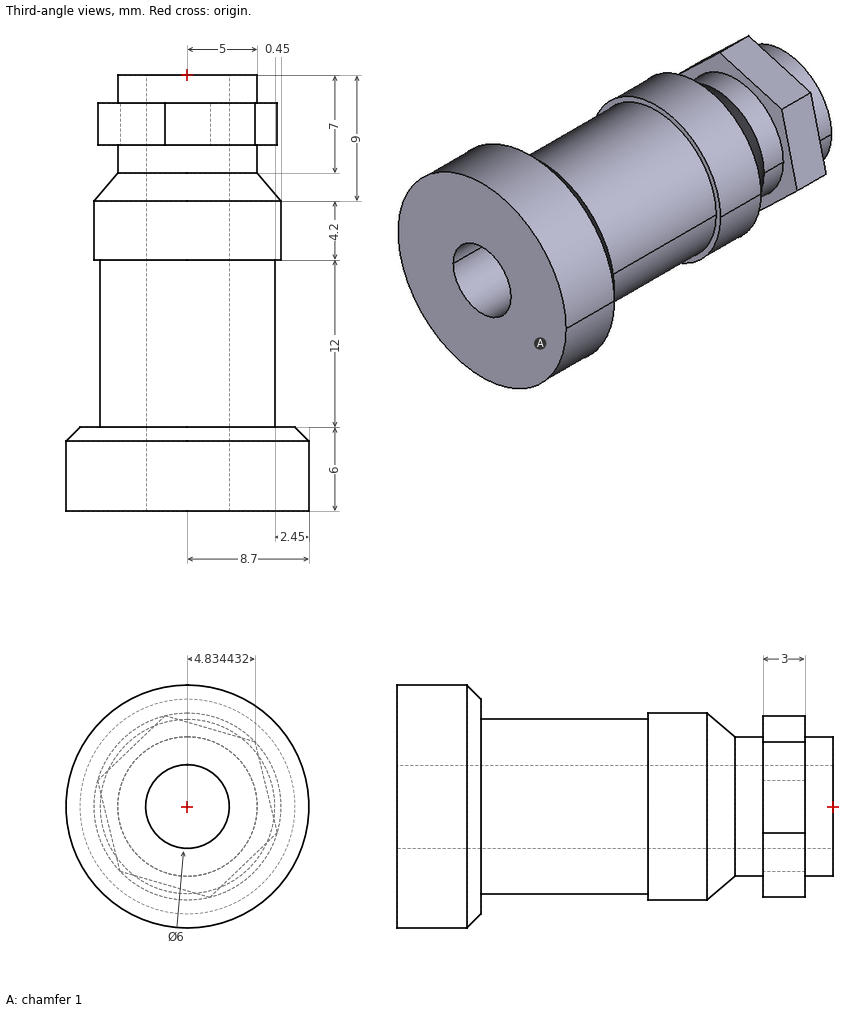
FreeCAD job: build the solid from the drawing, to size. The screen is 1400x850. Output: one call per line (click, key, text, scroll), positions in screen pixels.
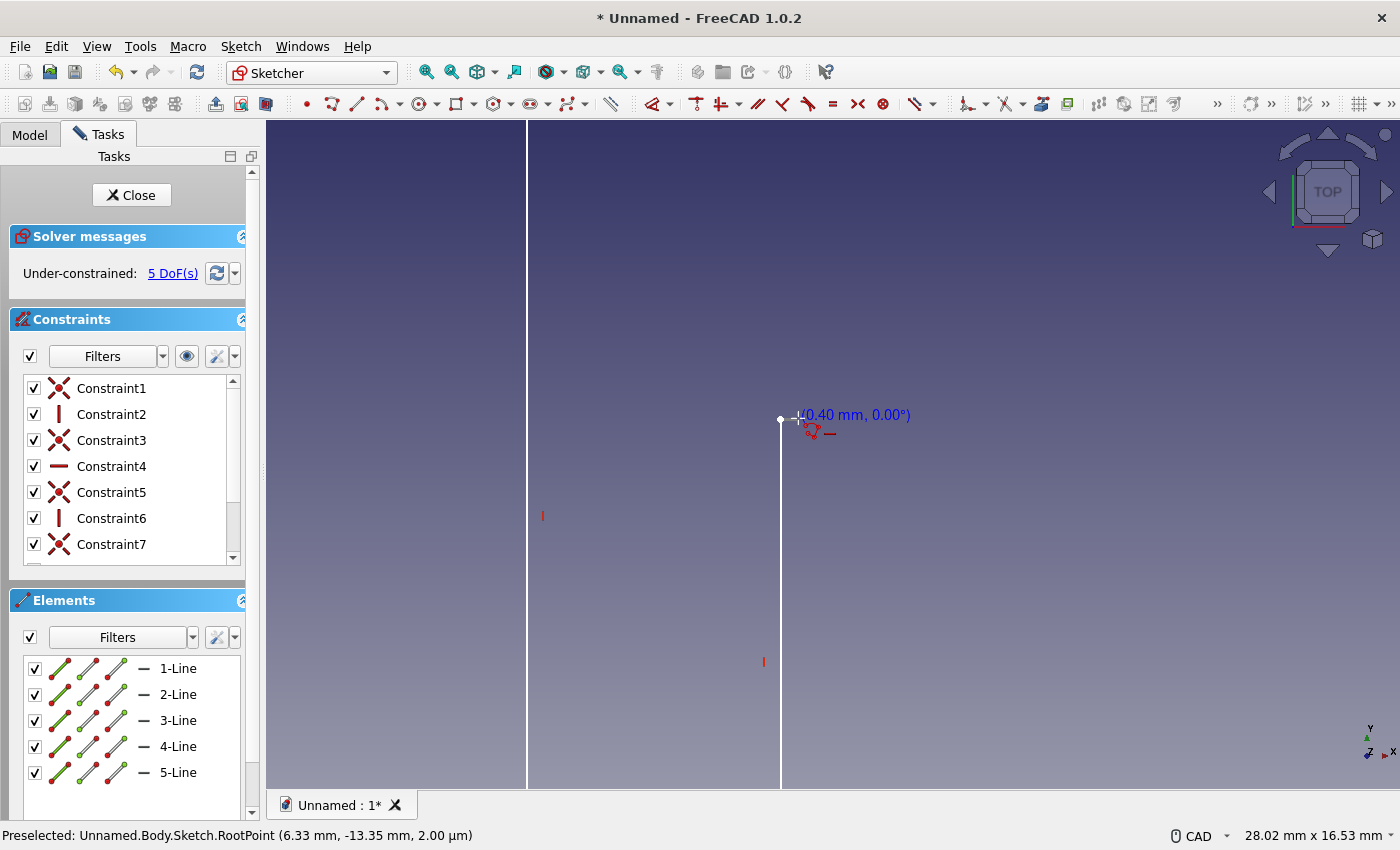
click(798, 417)
click(798, 247)
click(730, 166)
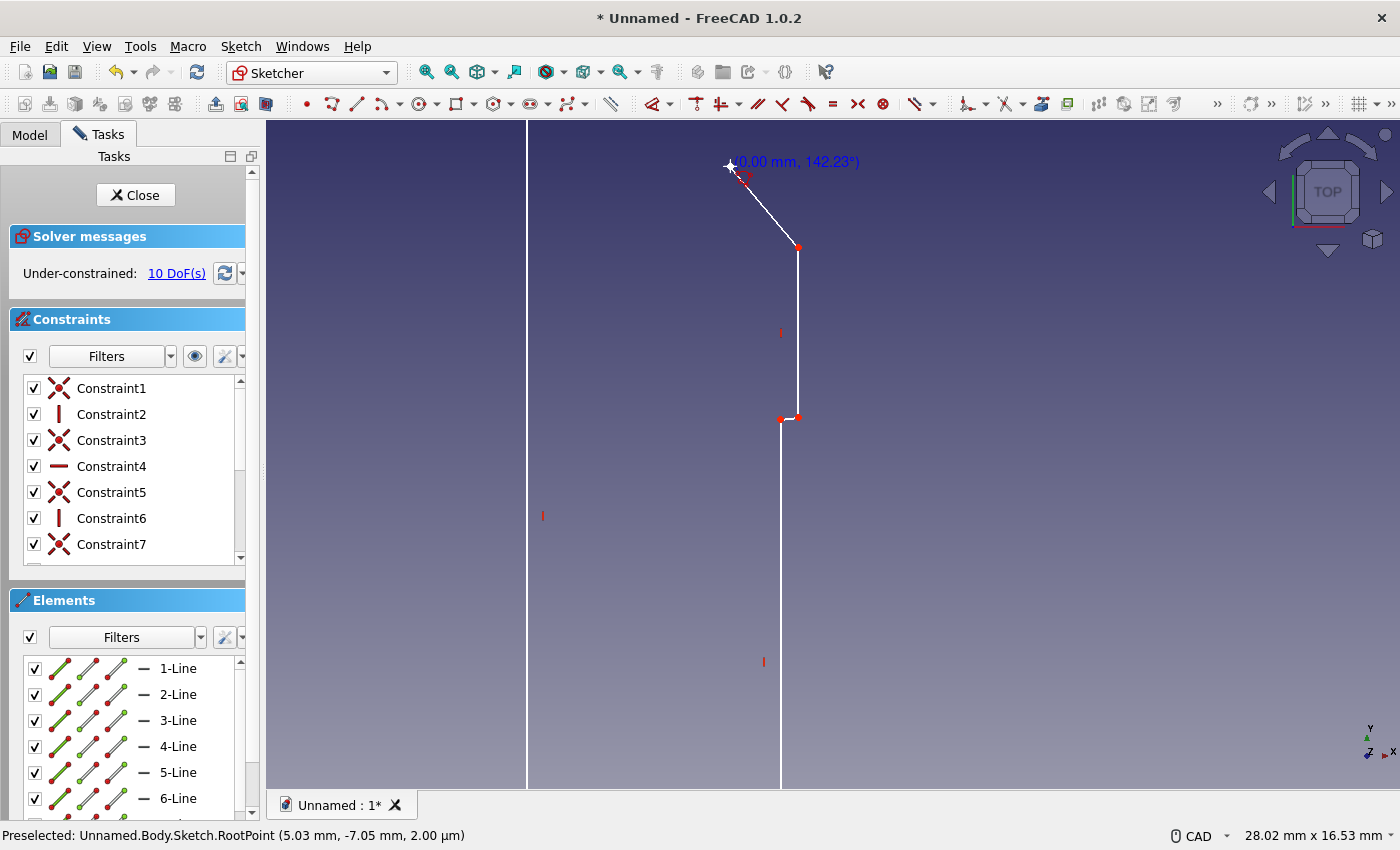
scroll(800, 420, down, 5)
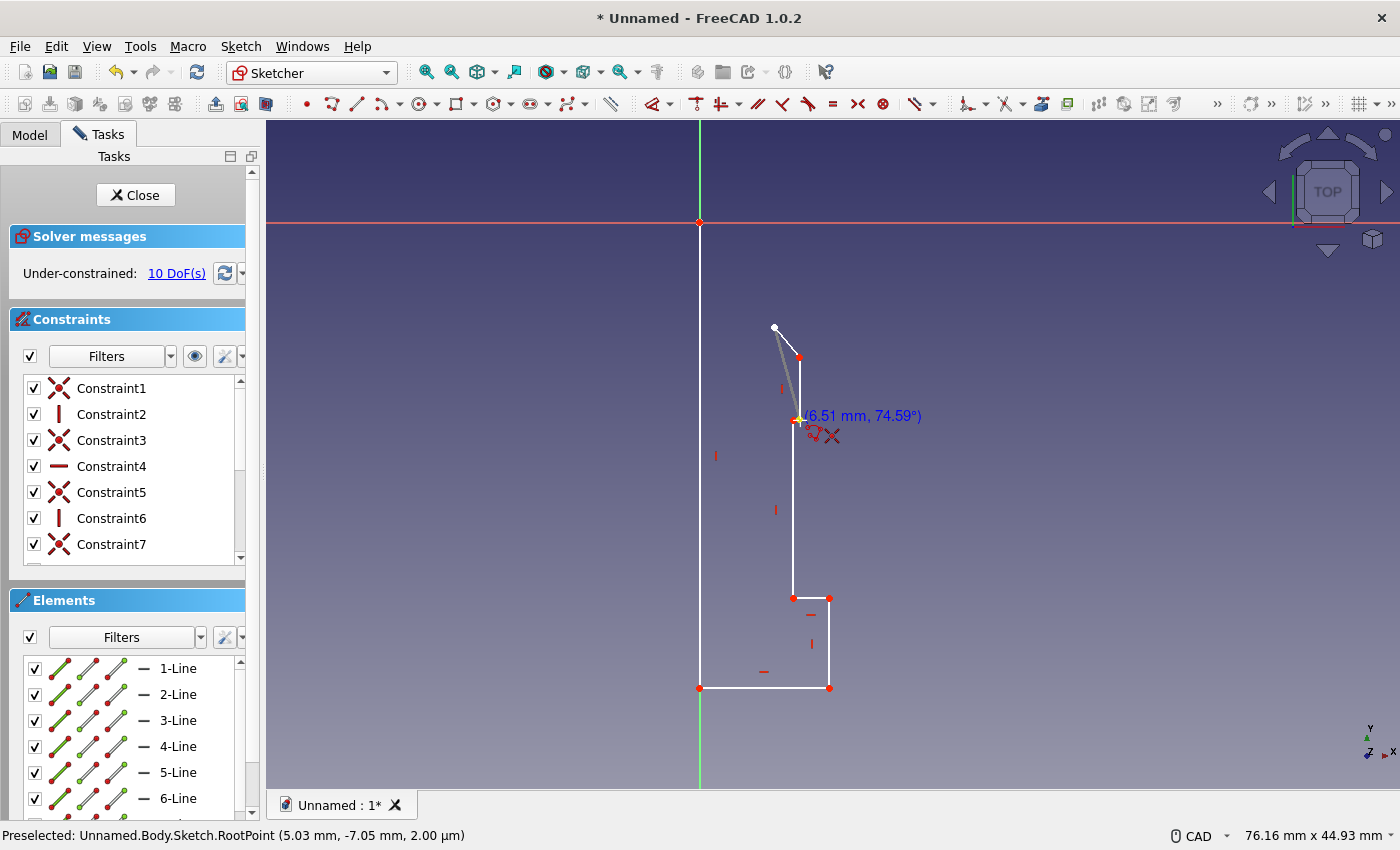
click(775, 232)
click(700, 223)
key(Escape)
key(Escape)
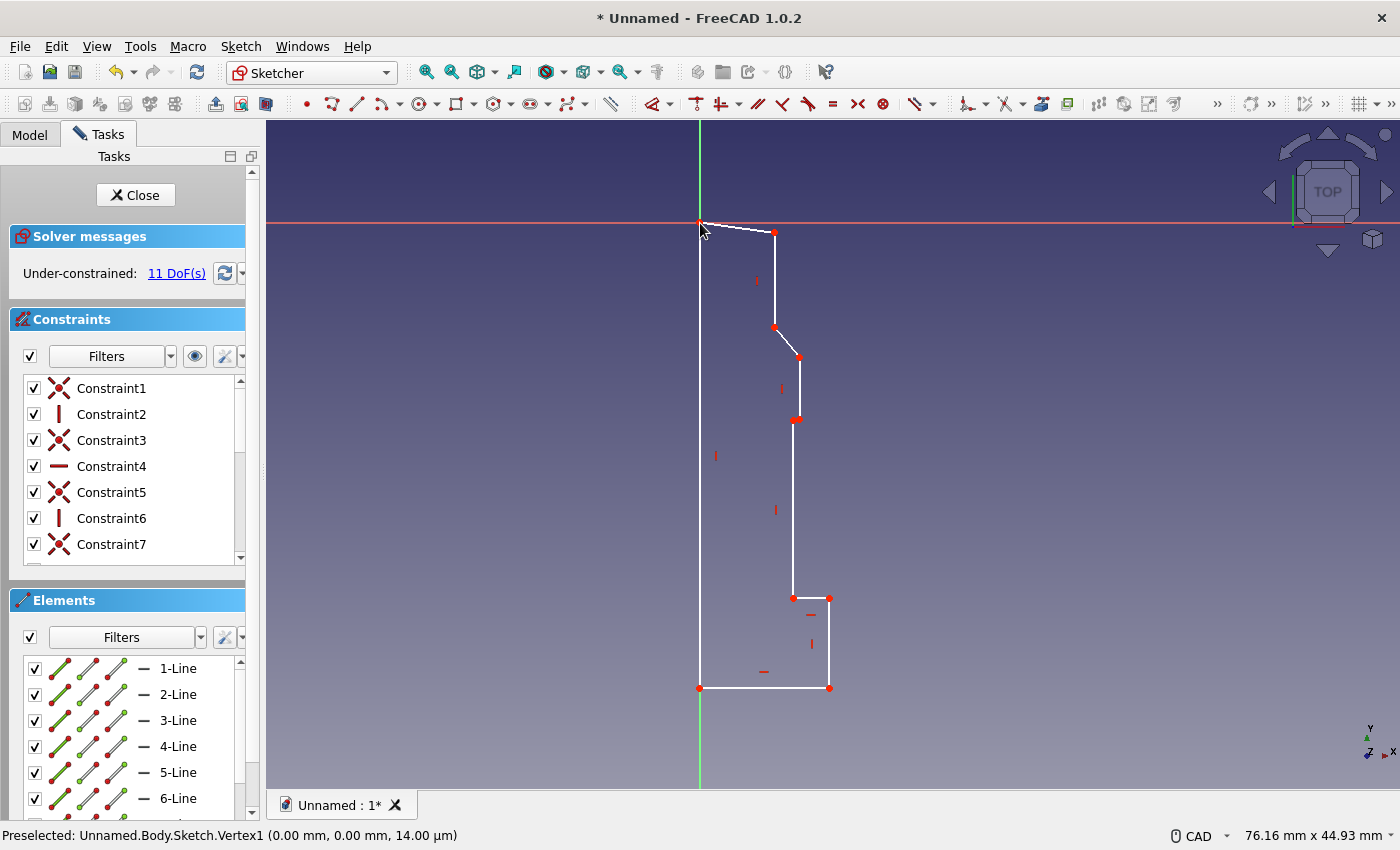
scroll(796, 420, up, 8)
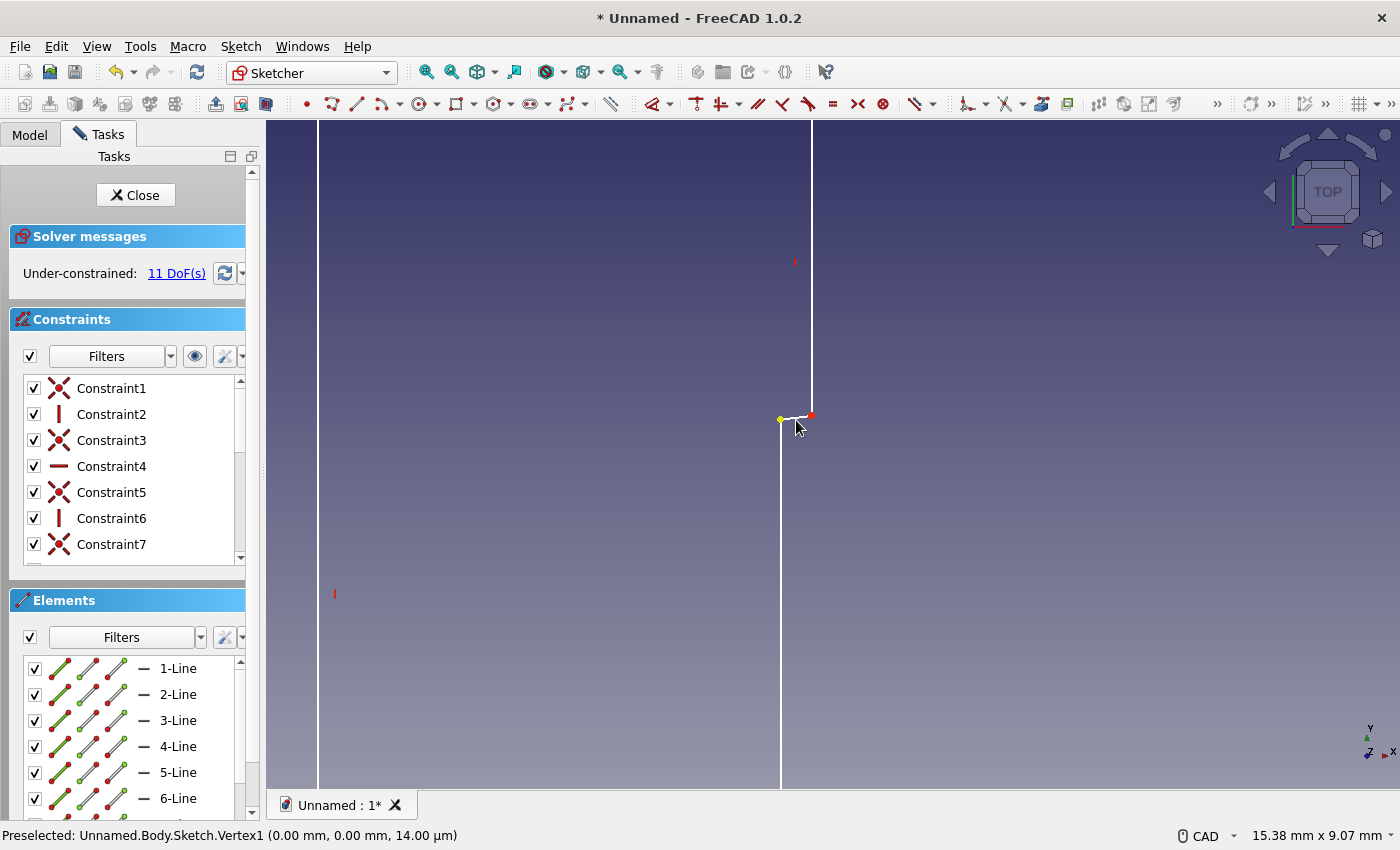
click(796, 418)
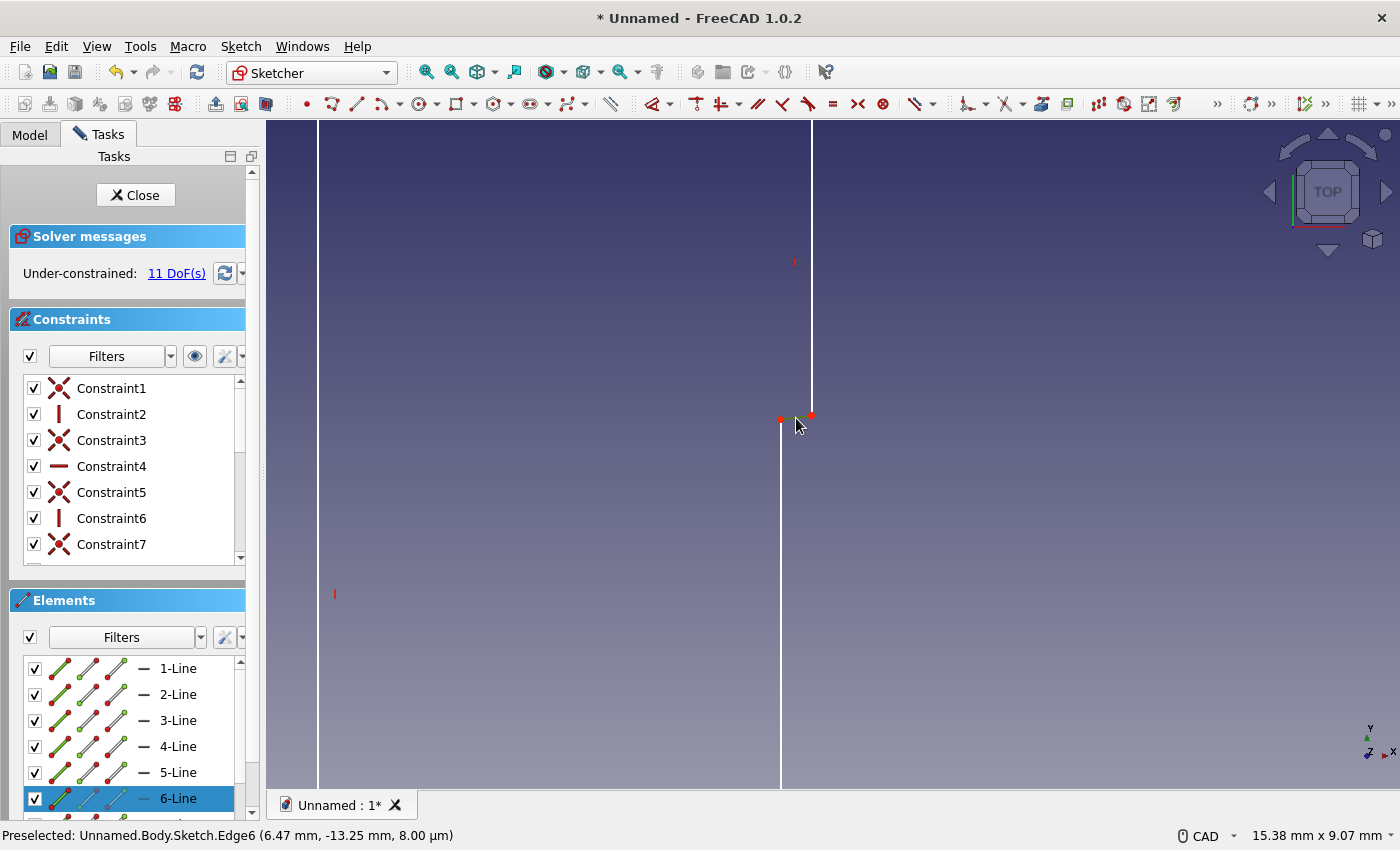
key(h)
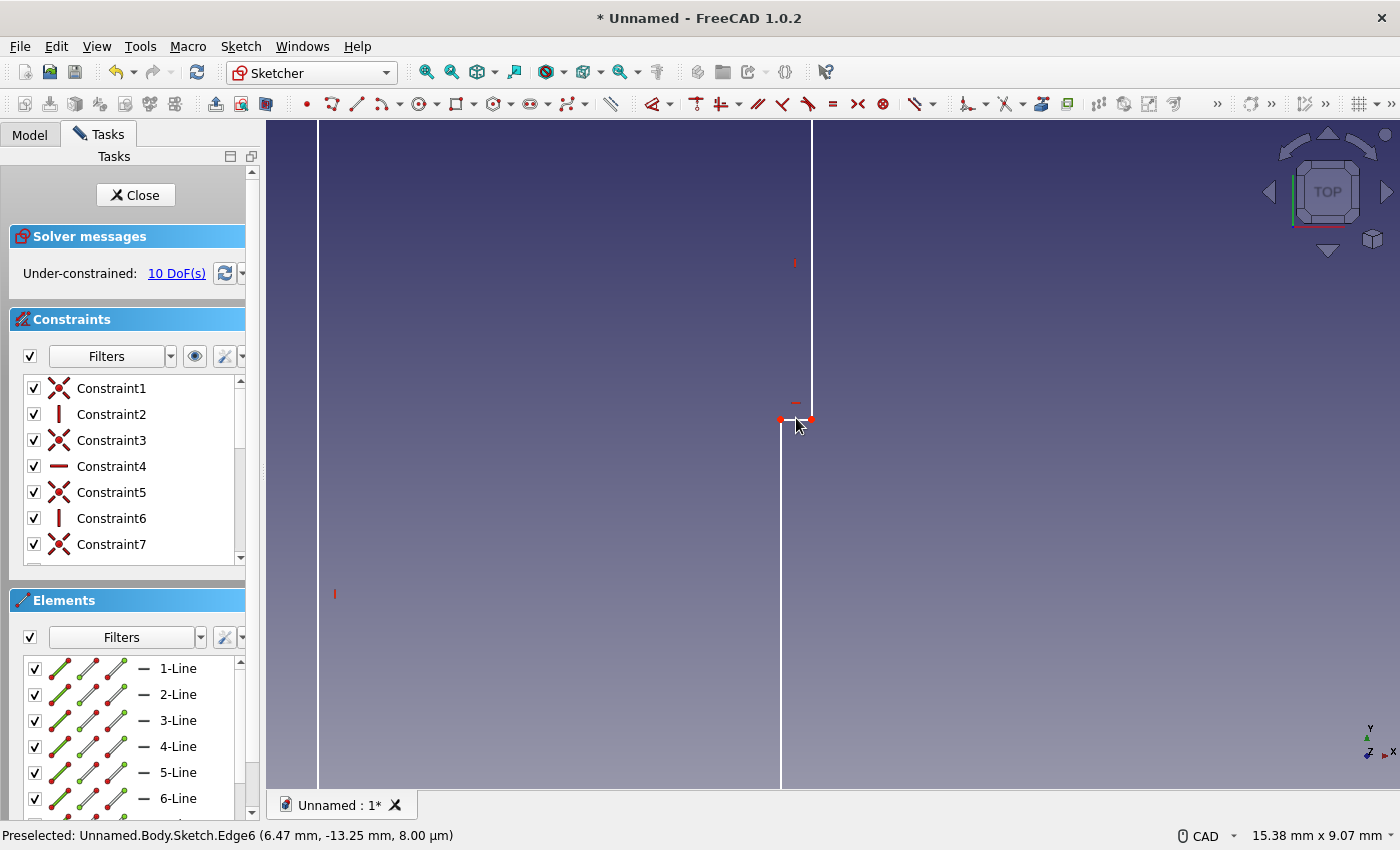
scroll(796, 420, down, 8)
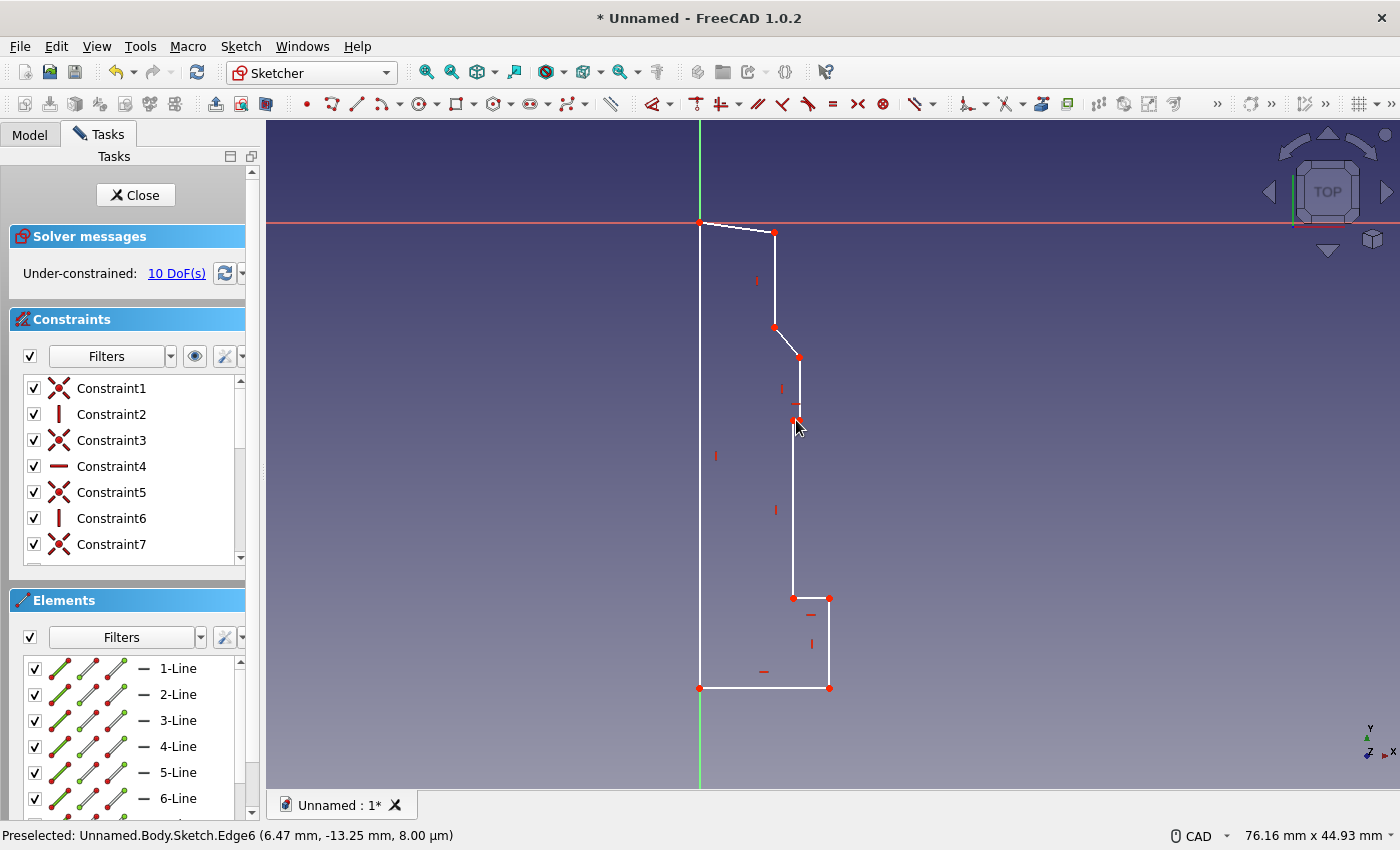
scroll(752, 230, up, 4)